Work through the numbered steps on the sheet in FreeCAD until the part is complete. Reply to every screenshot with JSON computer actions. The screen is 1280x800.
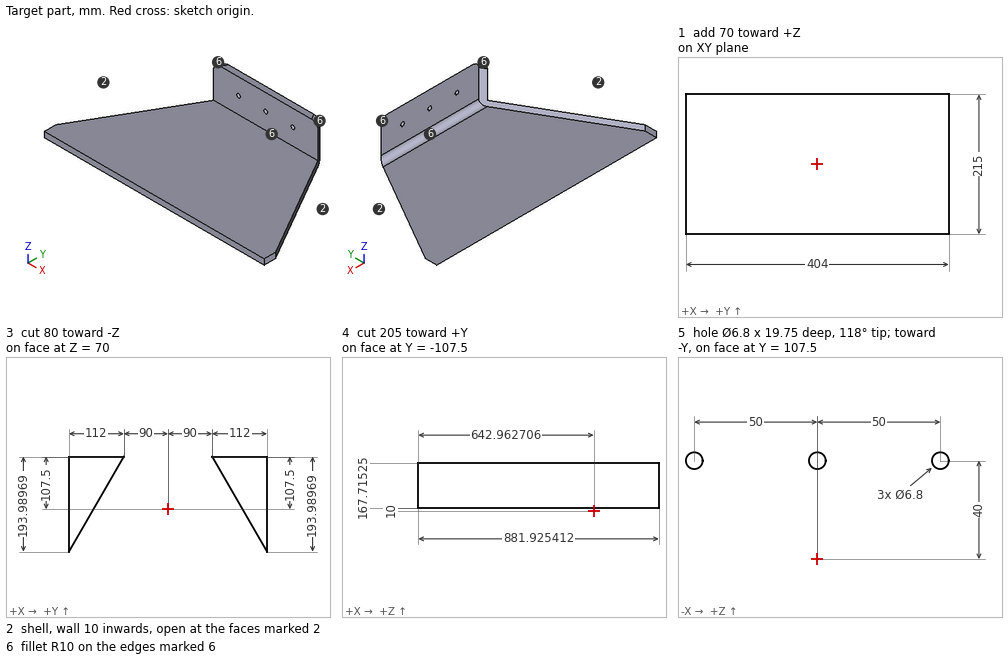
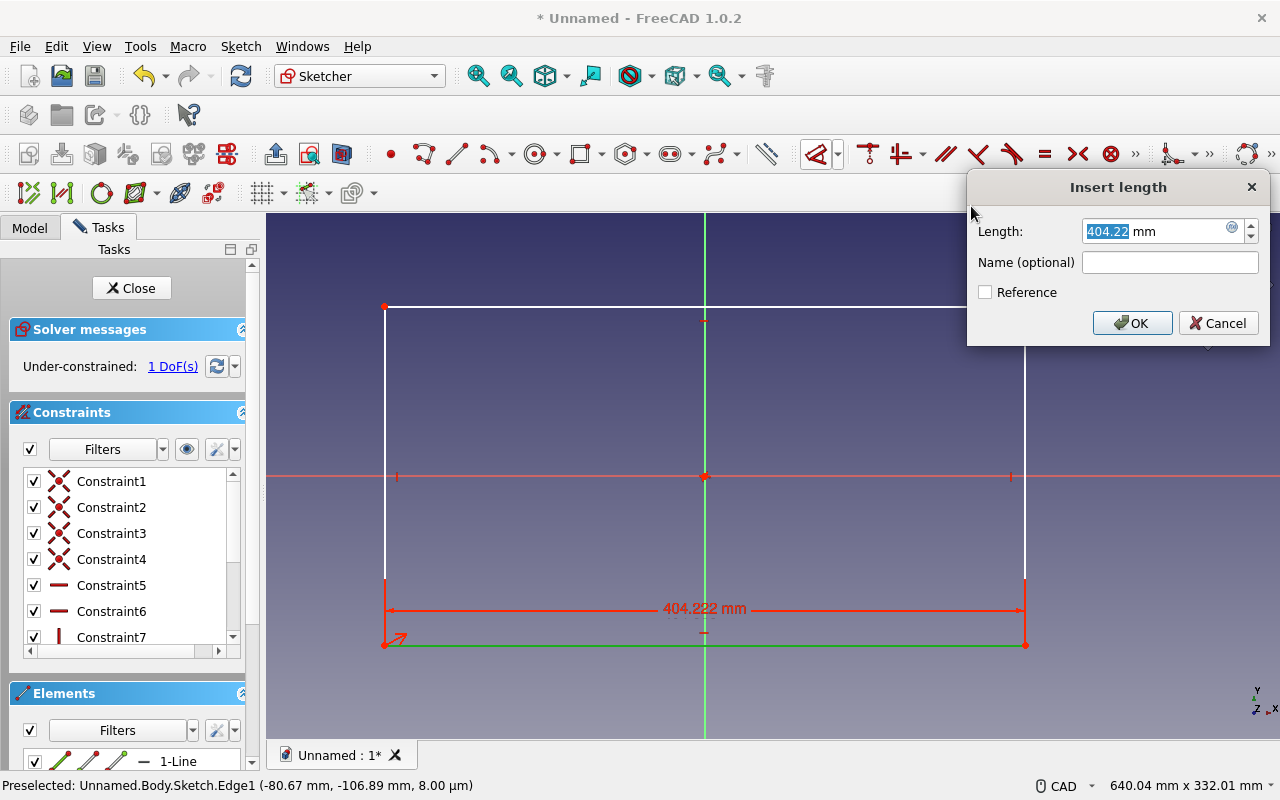
{"action": "type", "text": "404"}
{"action": "key", "text": "Return"}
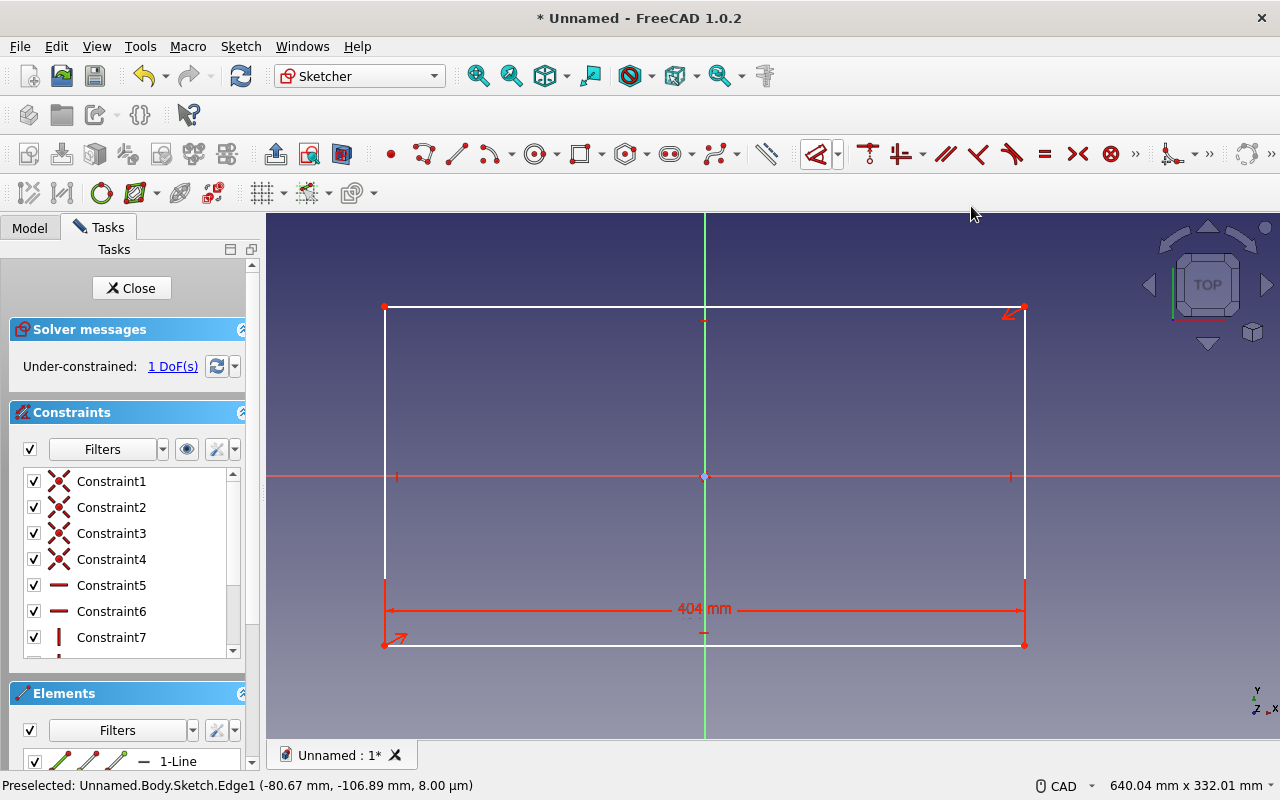
{"action": "left_click", "coordinate": [1025, 544]}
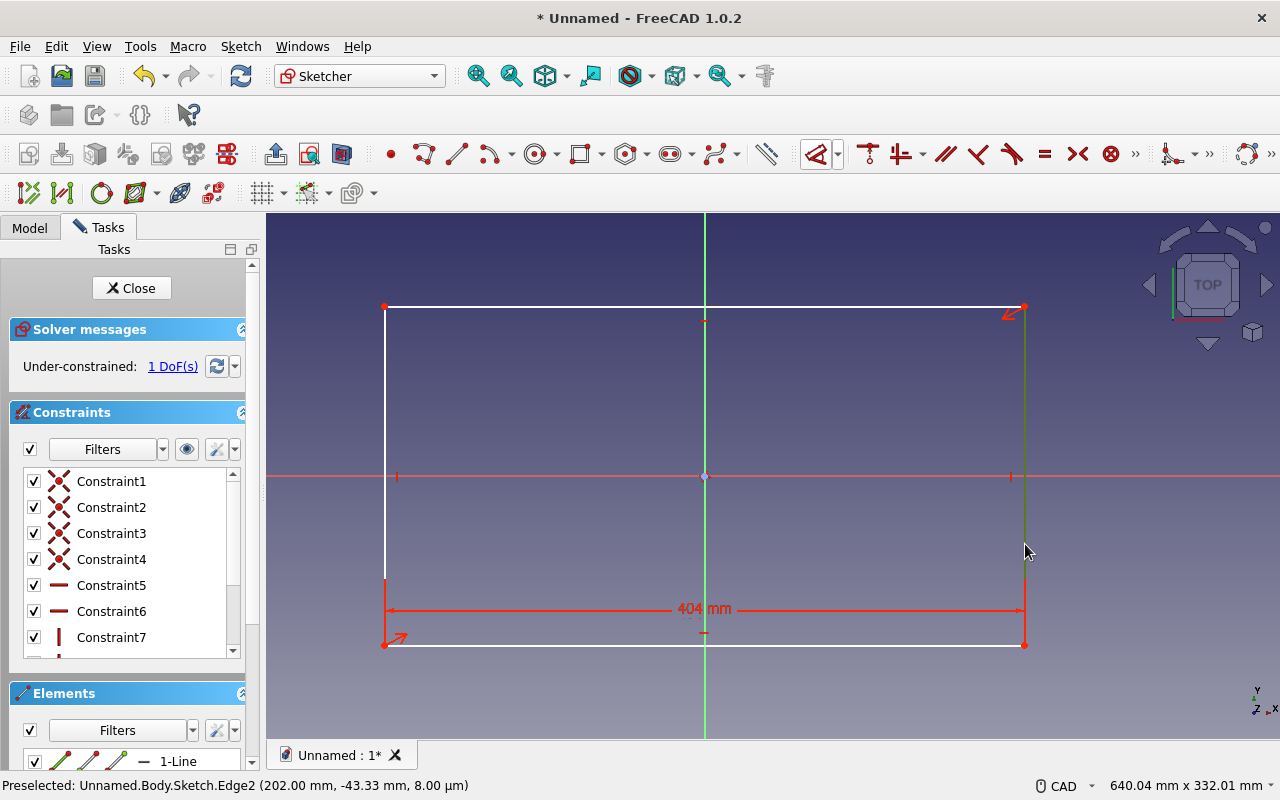
{"action": "left_click", "coordinate": [838, 154]}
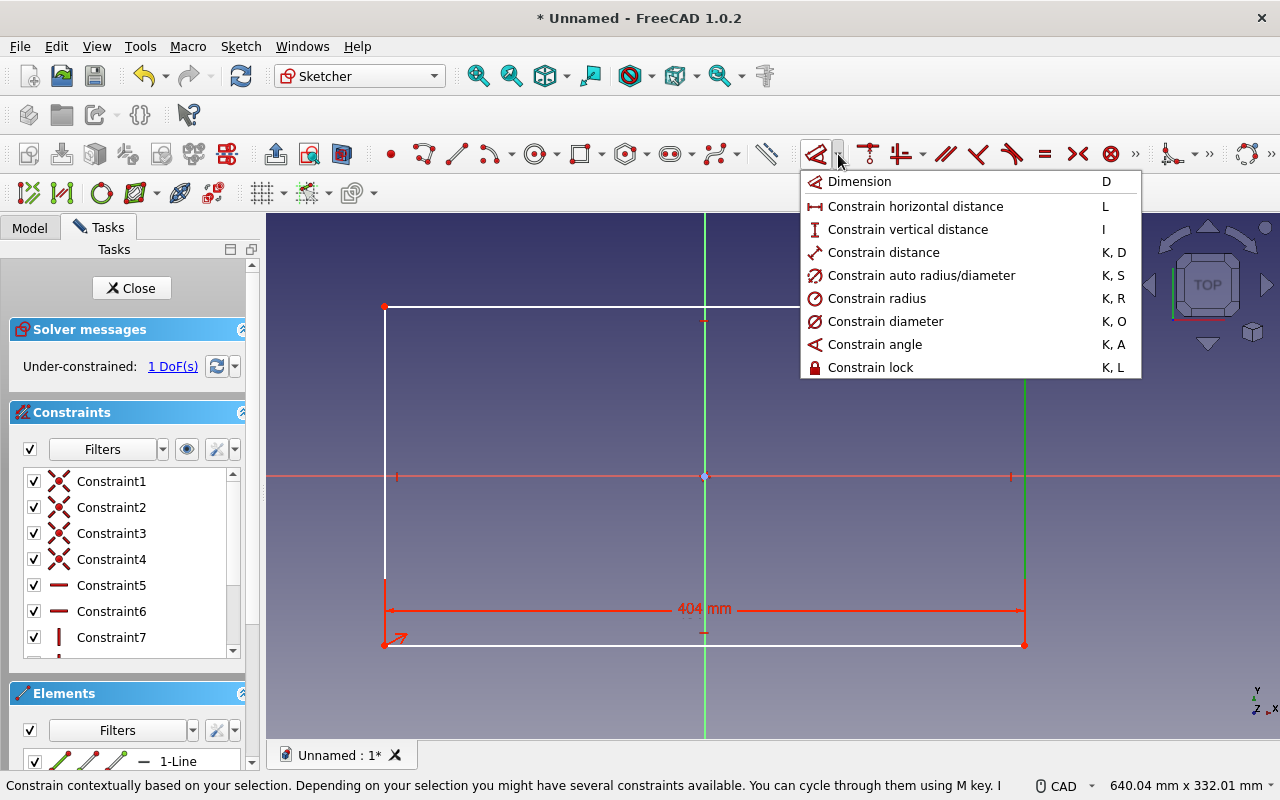
{"action": "left_click", "coordinate": [971, 230]}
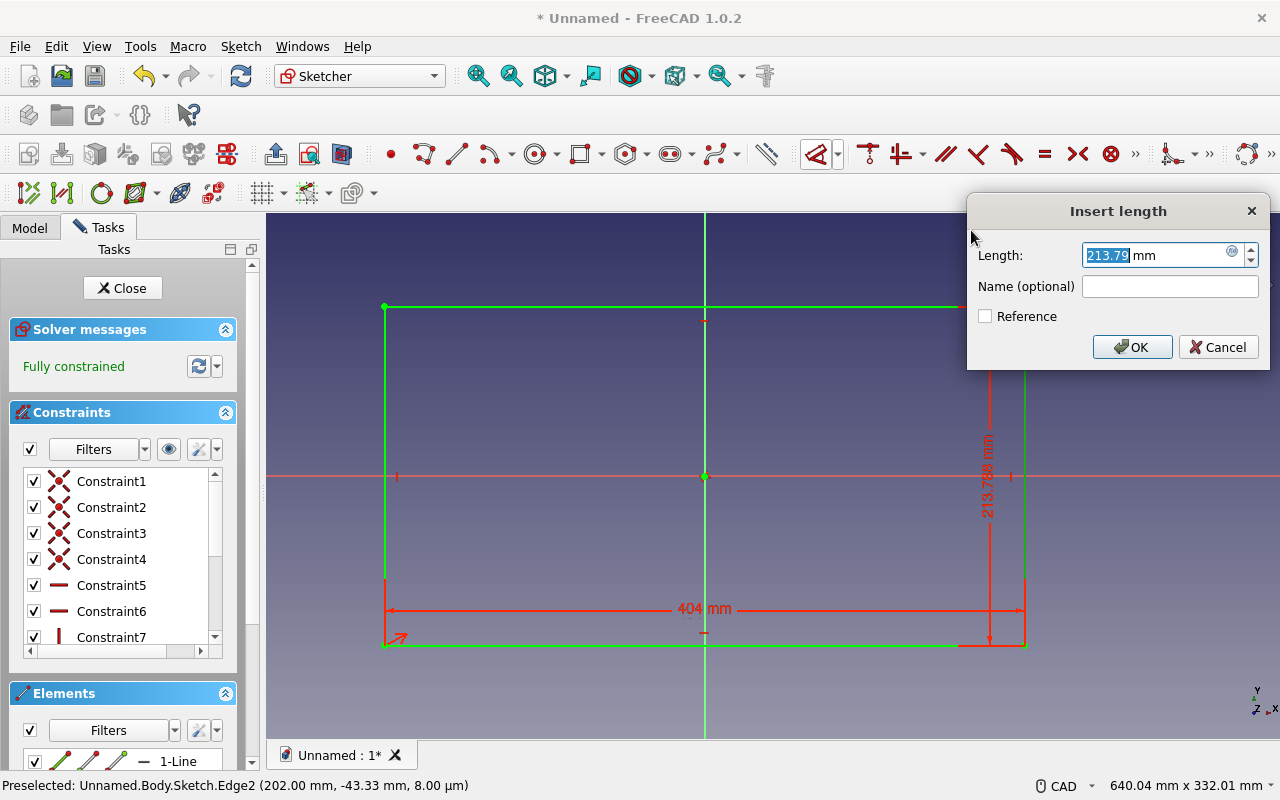
{"action": "type", "text": "215"}
{"action": "key", "text": "Return"}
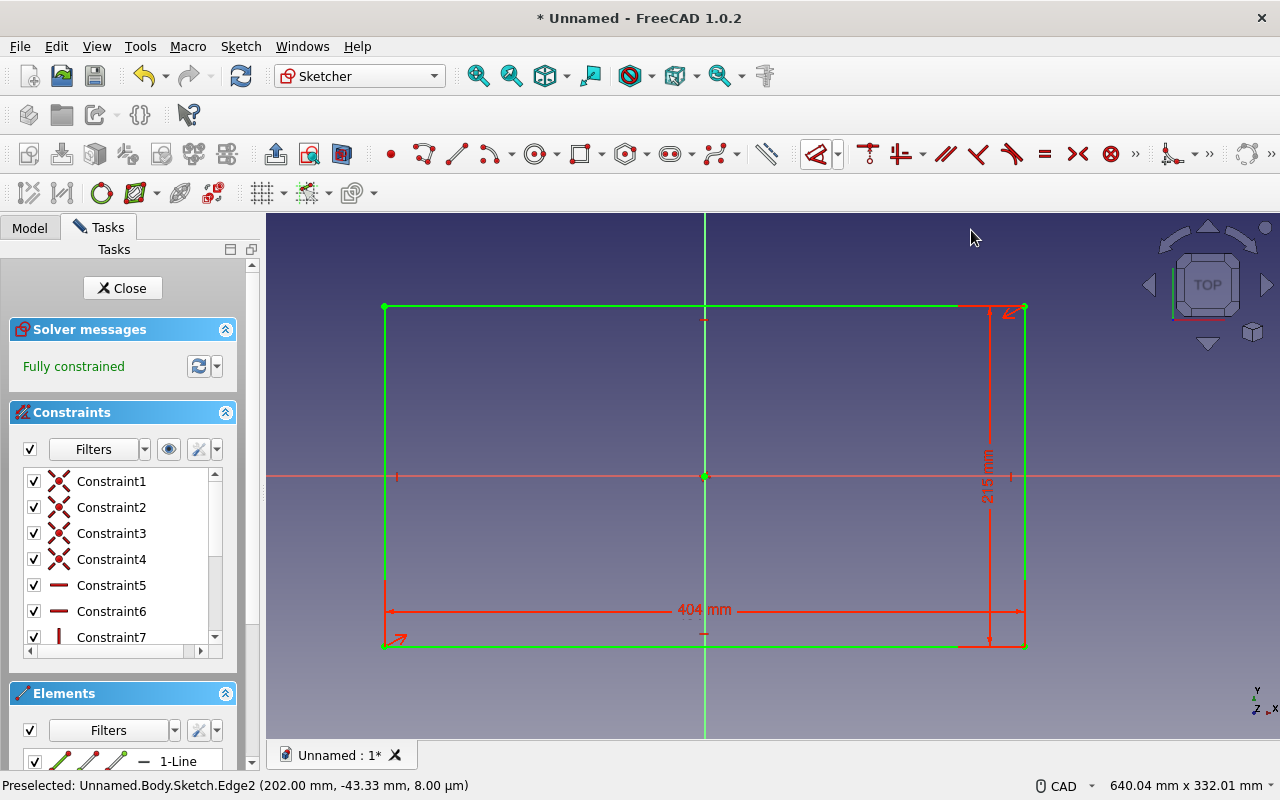
{"action": "left_click", "coordinate": [123, 288]}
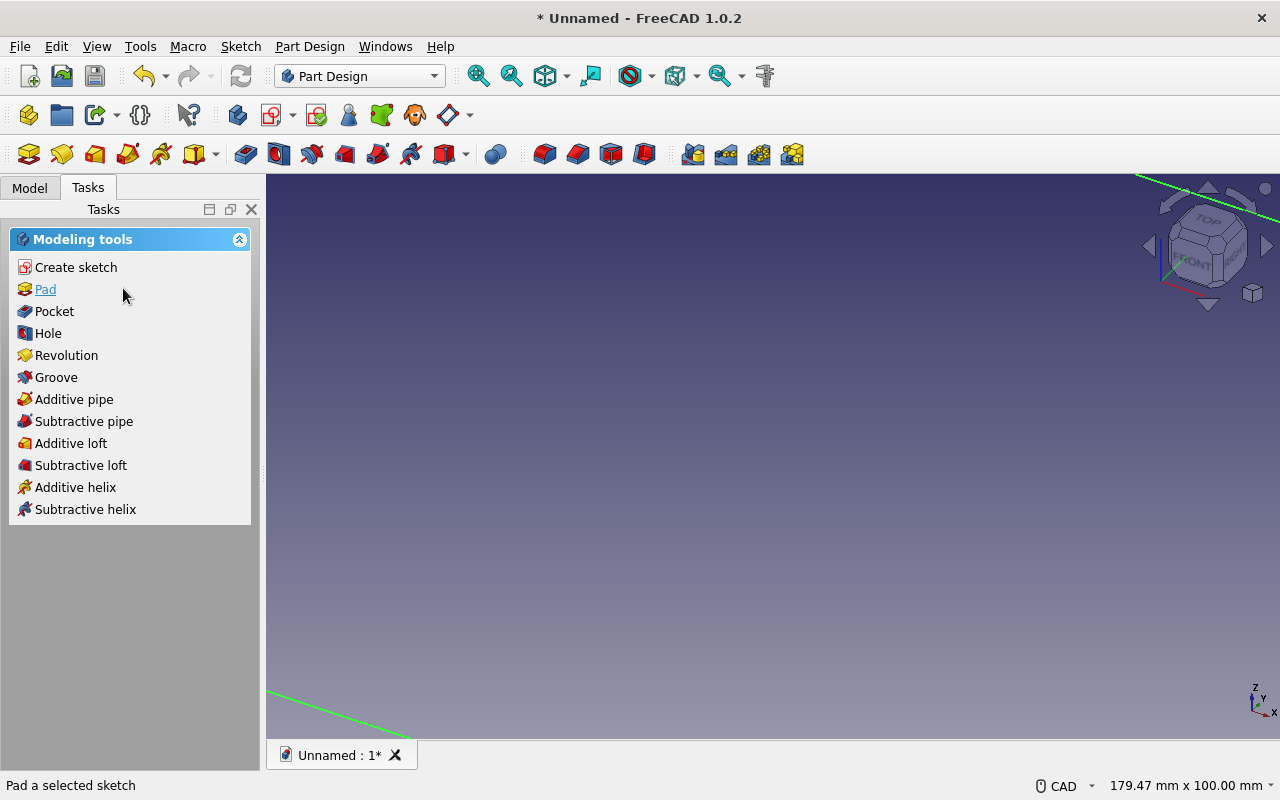
{"action": "left_click", "coordinate": [29, 154]}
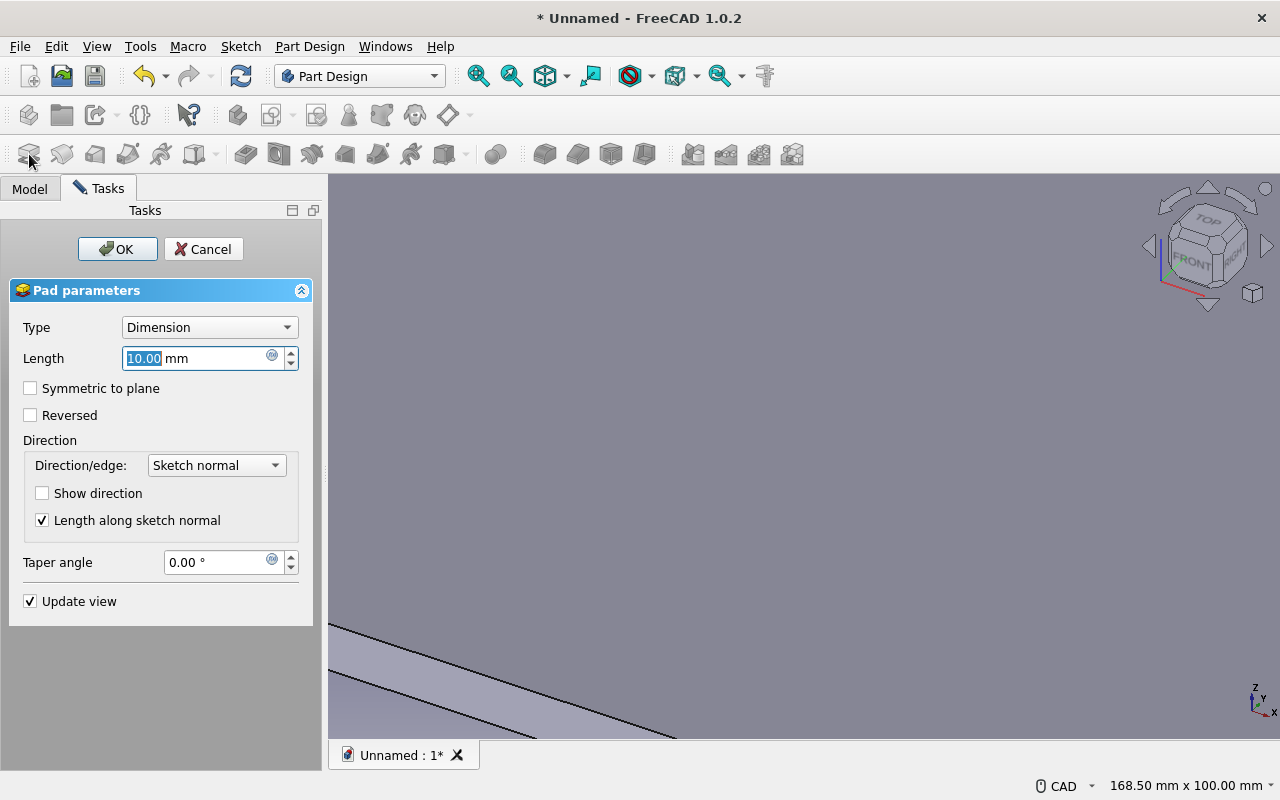
{"action": "type", "text": "70"}
{"action": "key", "text": "Tab"}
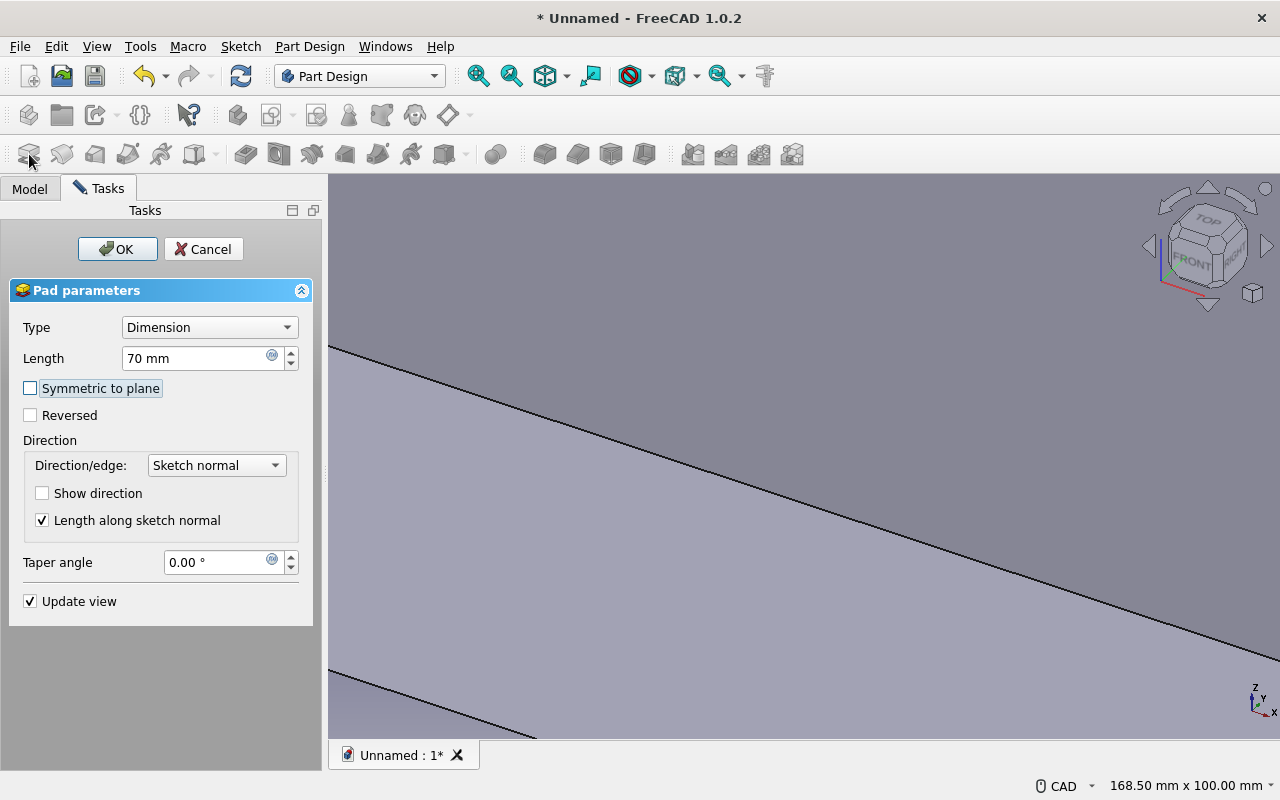
{"action": "left_click", "coordinate": [118, 249]}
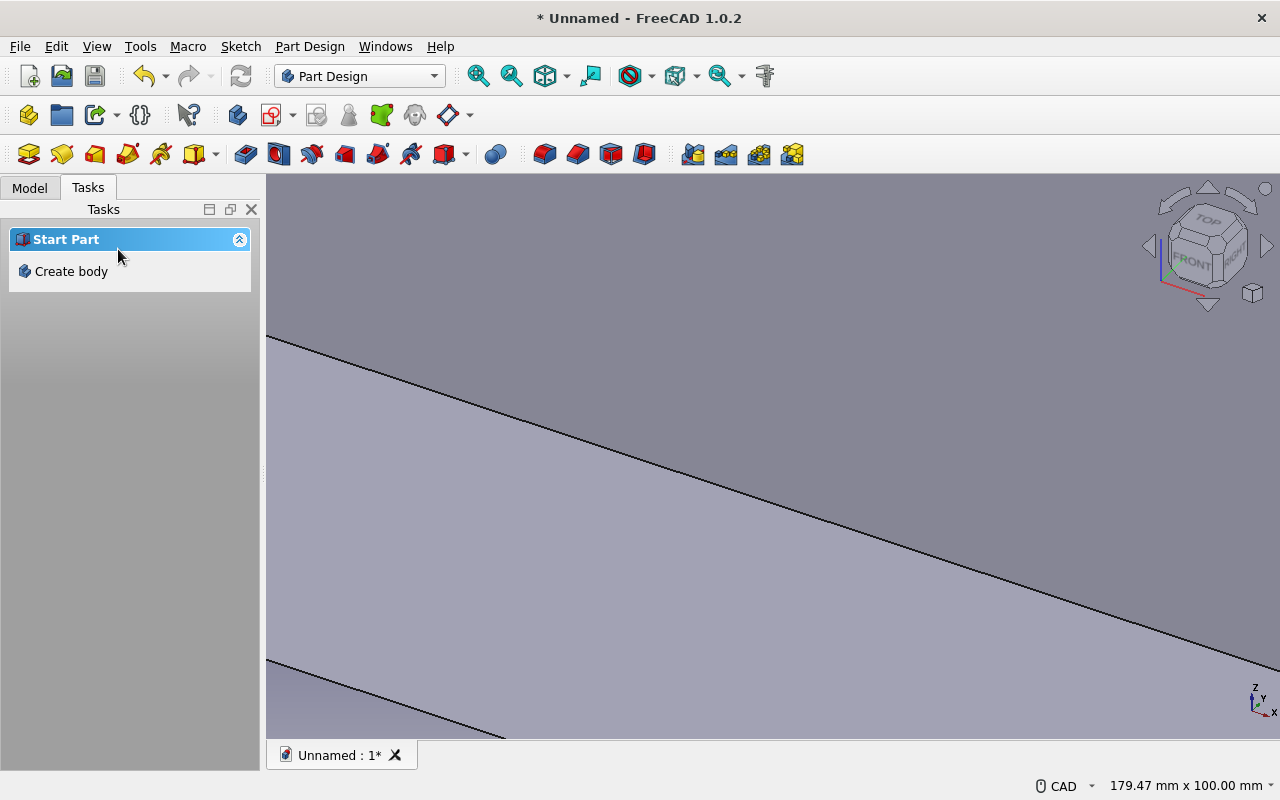
{"action": "left_click", "coordinate": [479, 76]}